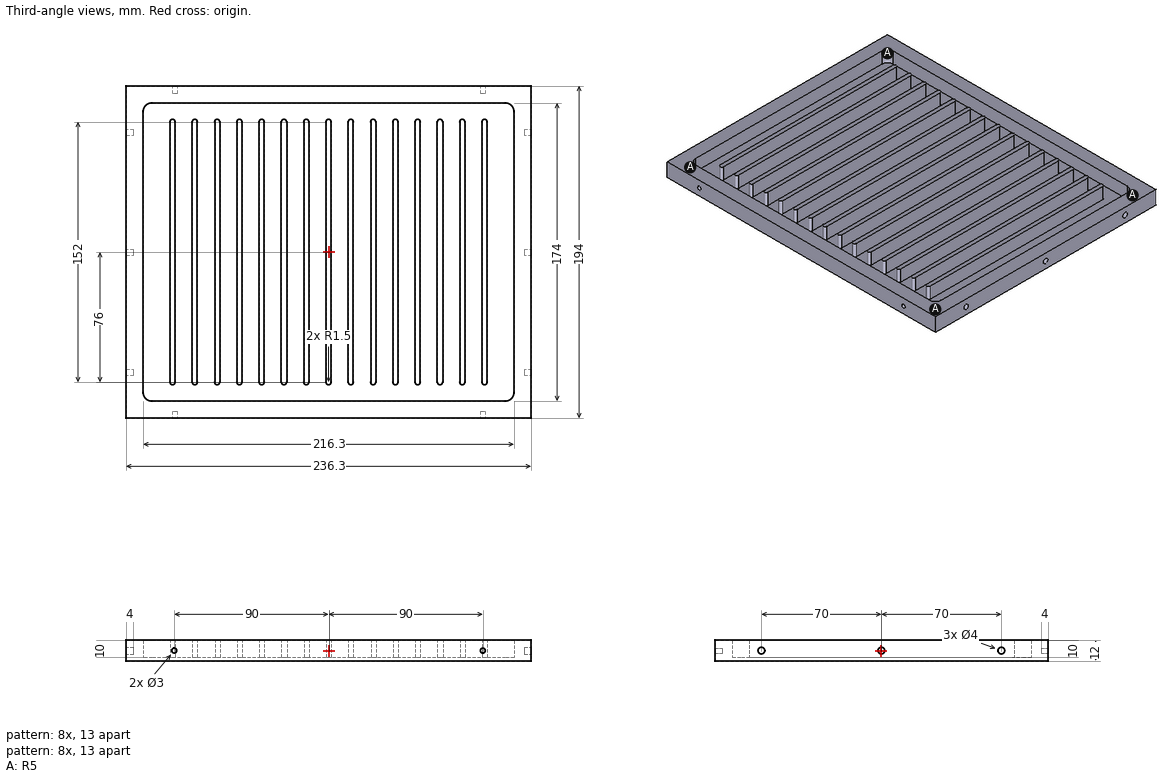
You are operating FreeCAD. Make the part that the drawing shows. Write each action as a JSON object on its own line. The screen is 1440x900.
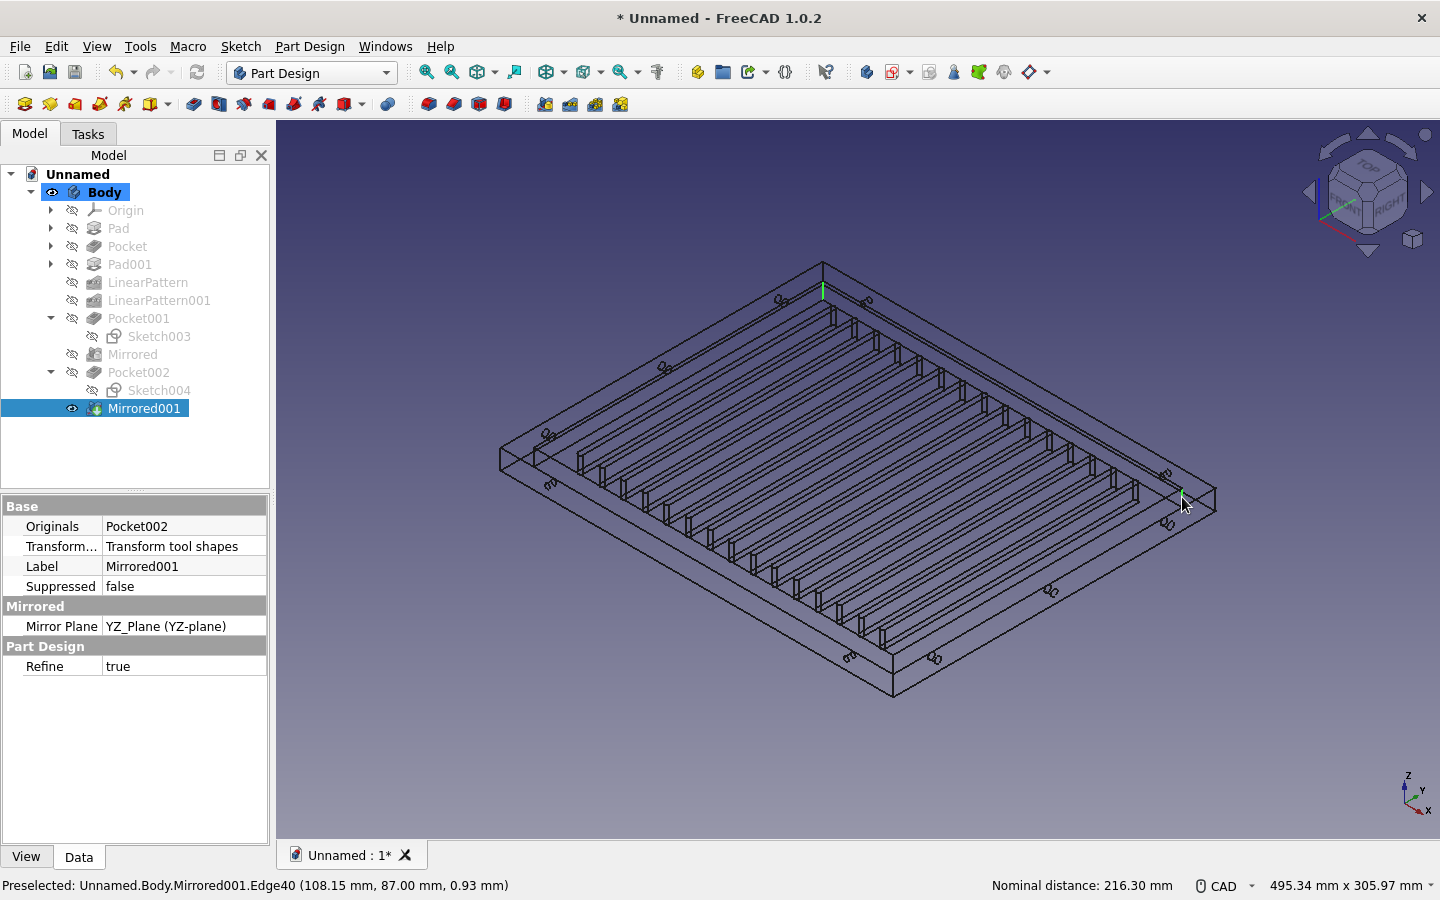
{"action": "left_click", "coordinate": [893, 664], "text": "ctrl"}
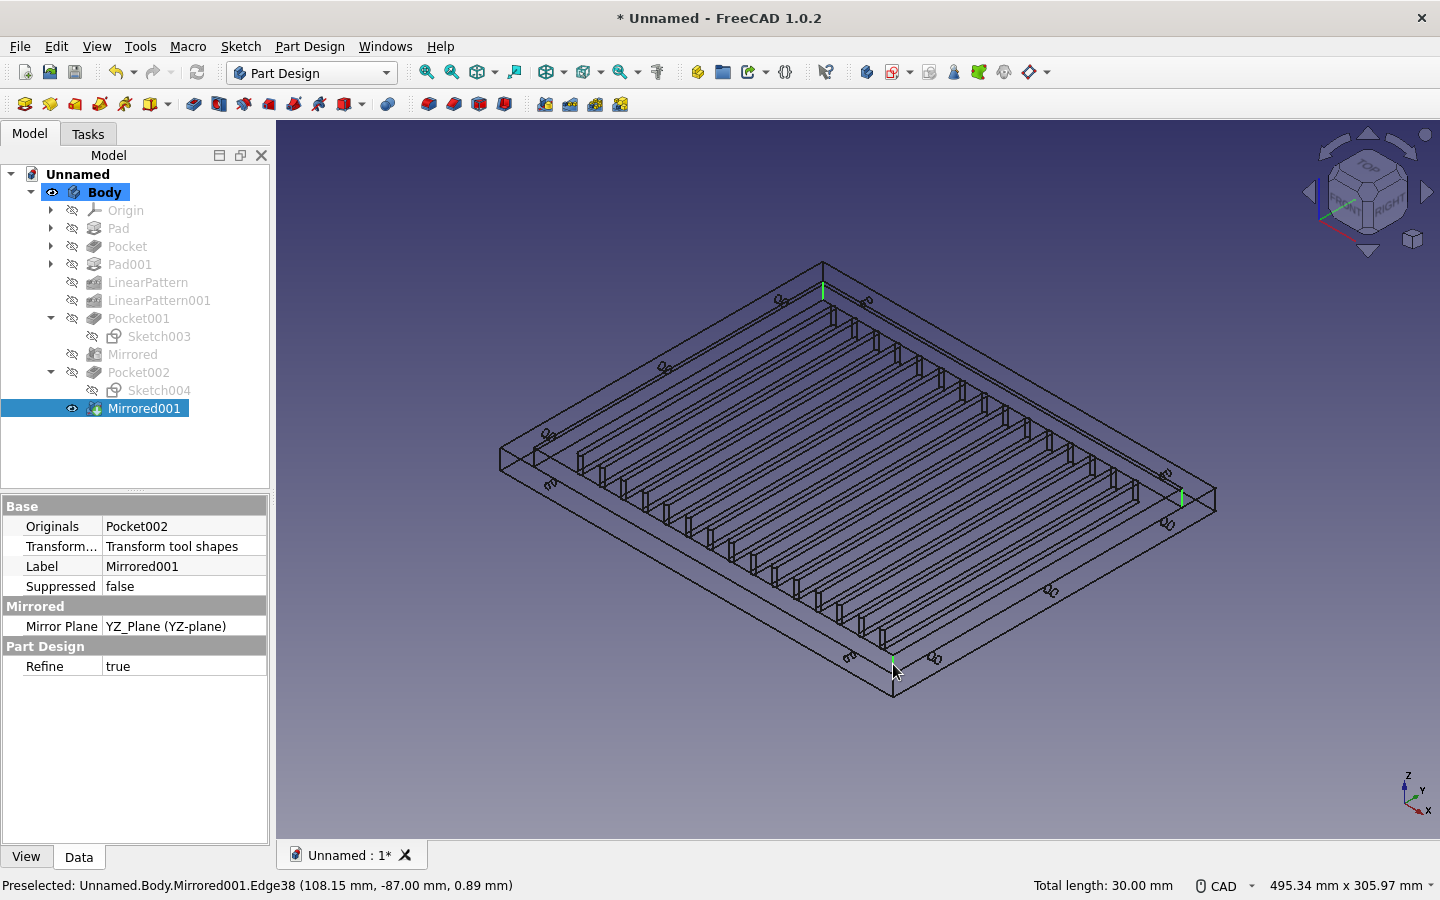
{"action": "left_click", "coordinate": [534, 456], "text": "ctrl"}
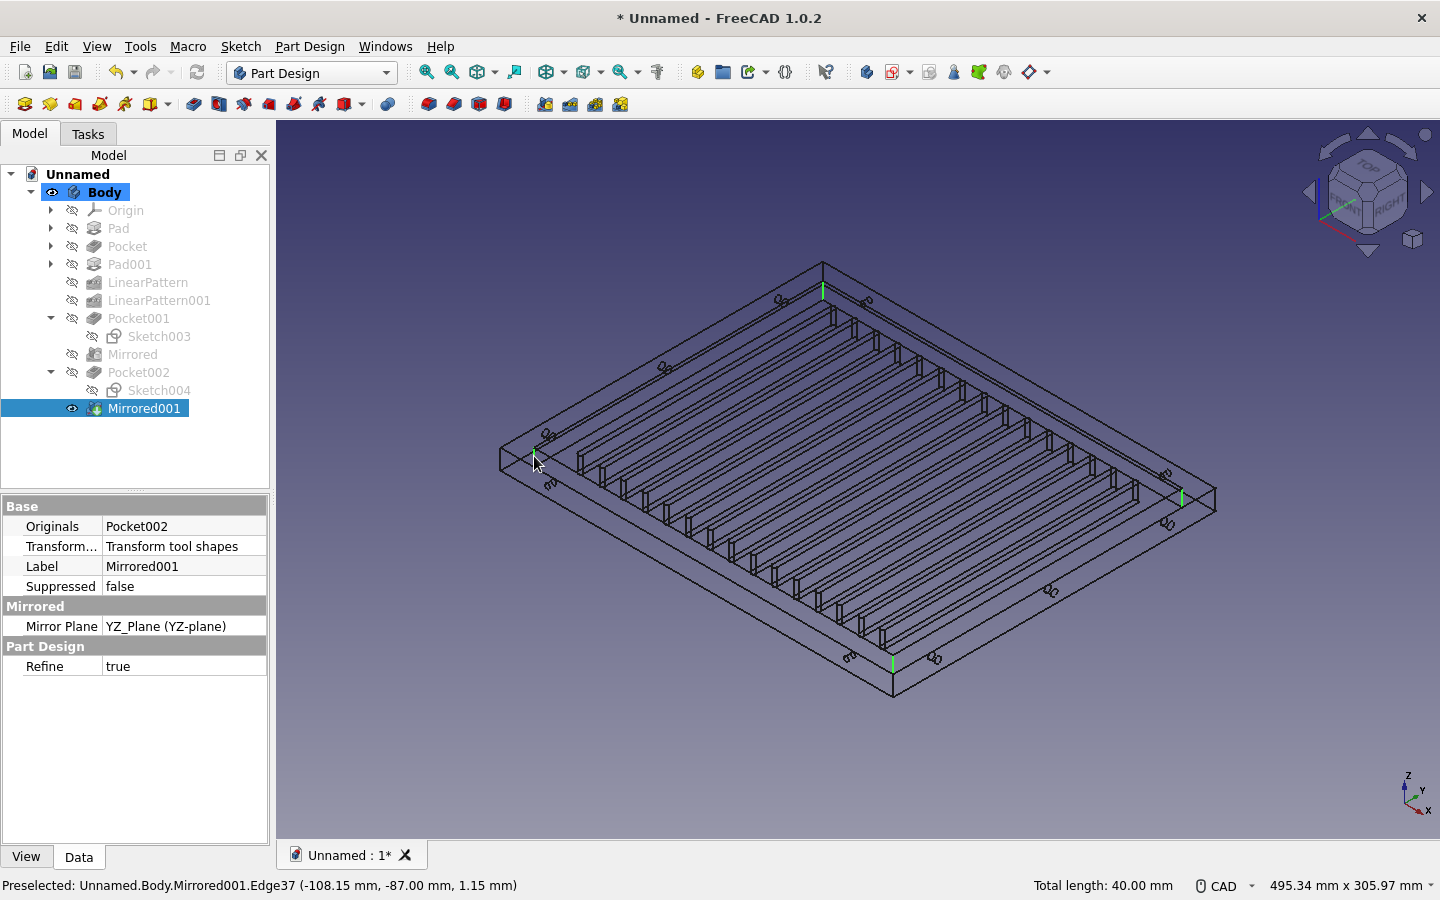
{"action": "key", "text": "v 1"}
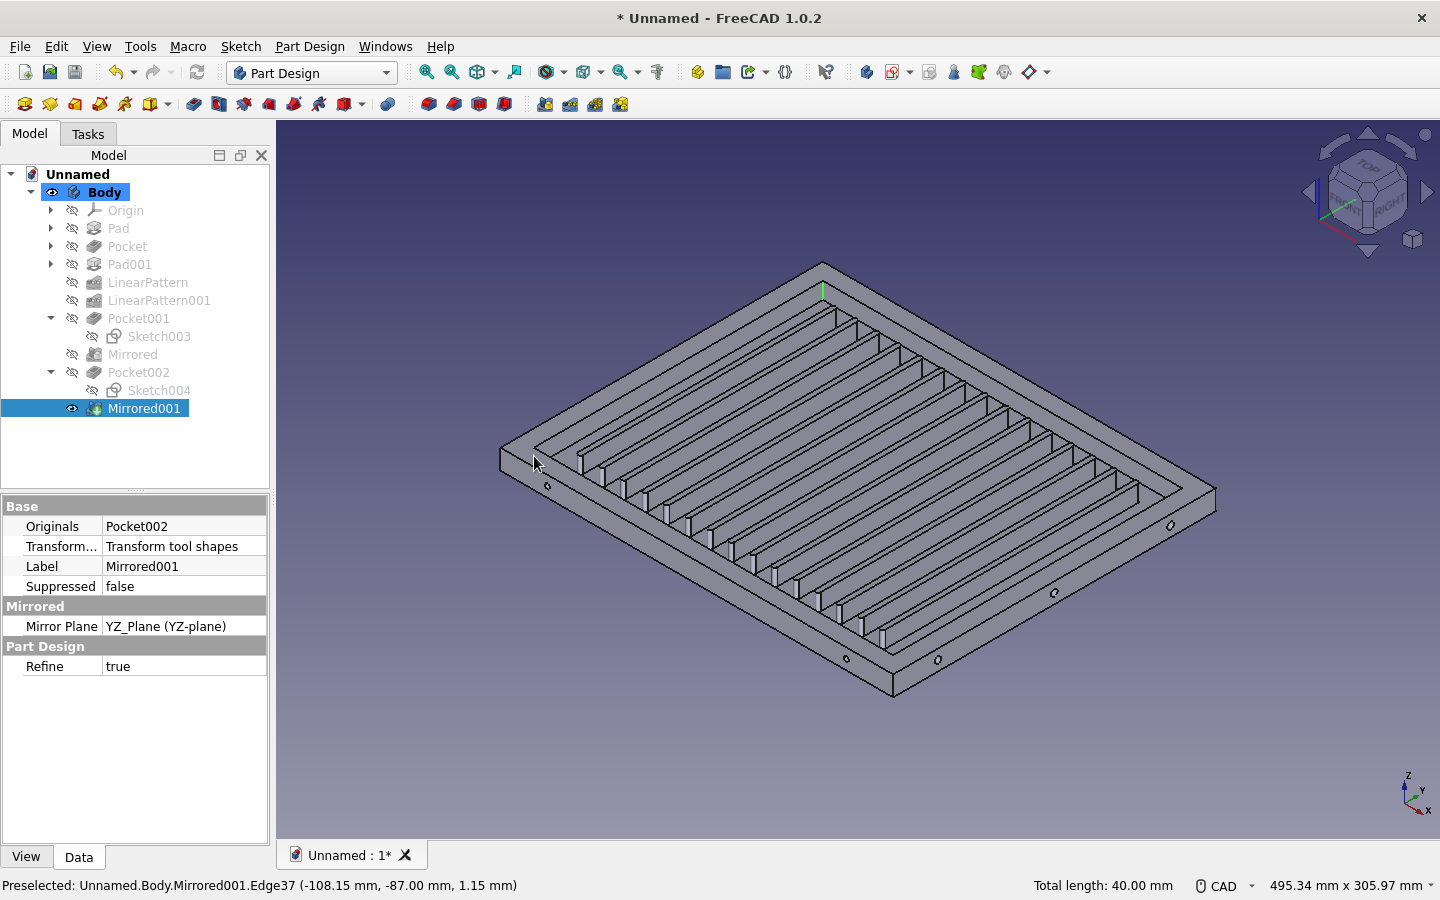
{"action": "left_click", "coordinate": [429, 104]}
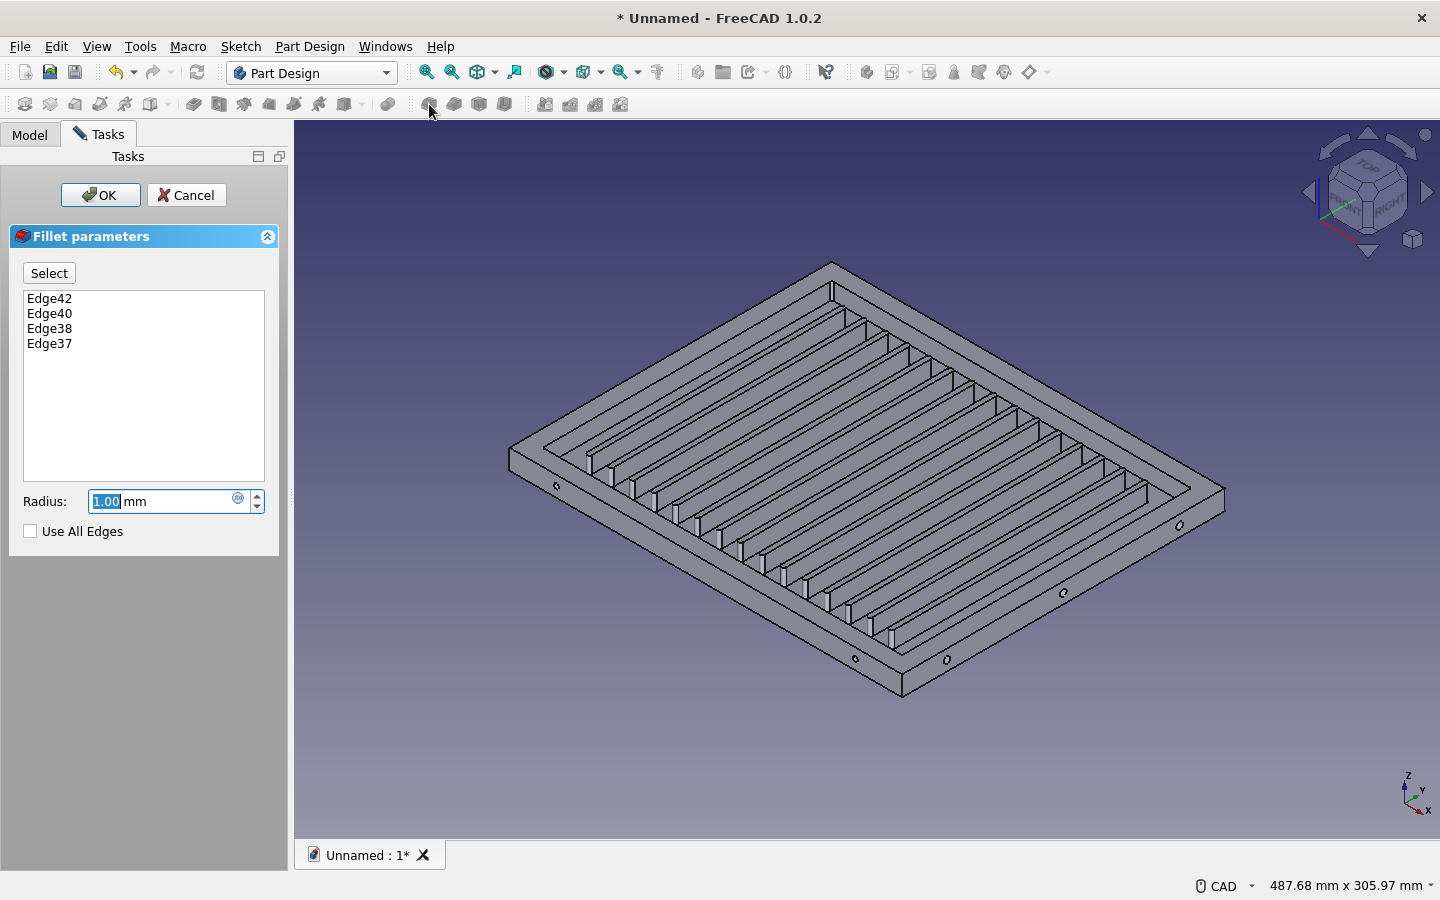
{"action": "type", "text": "5"}
{"action": "key", "text": "Tab"}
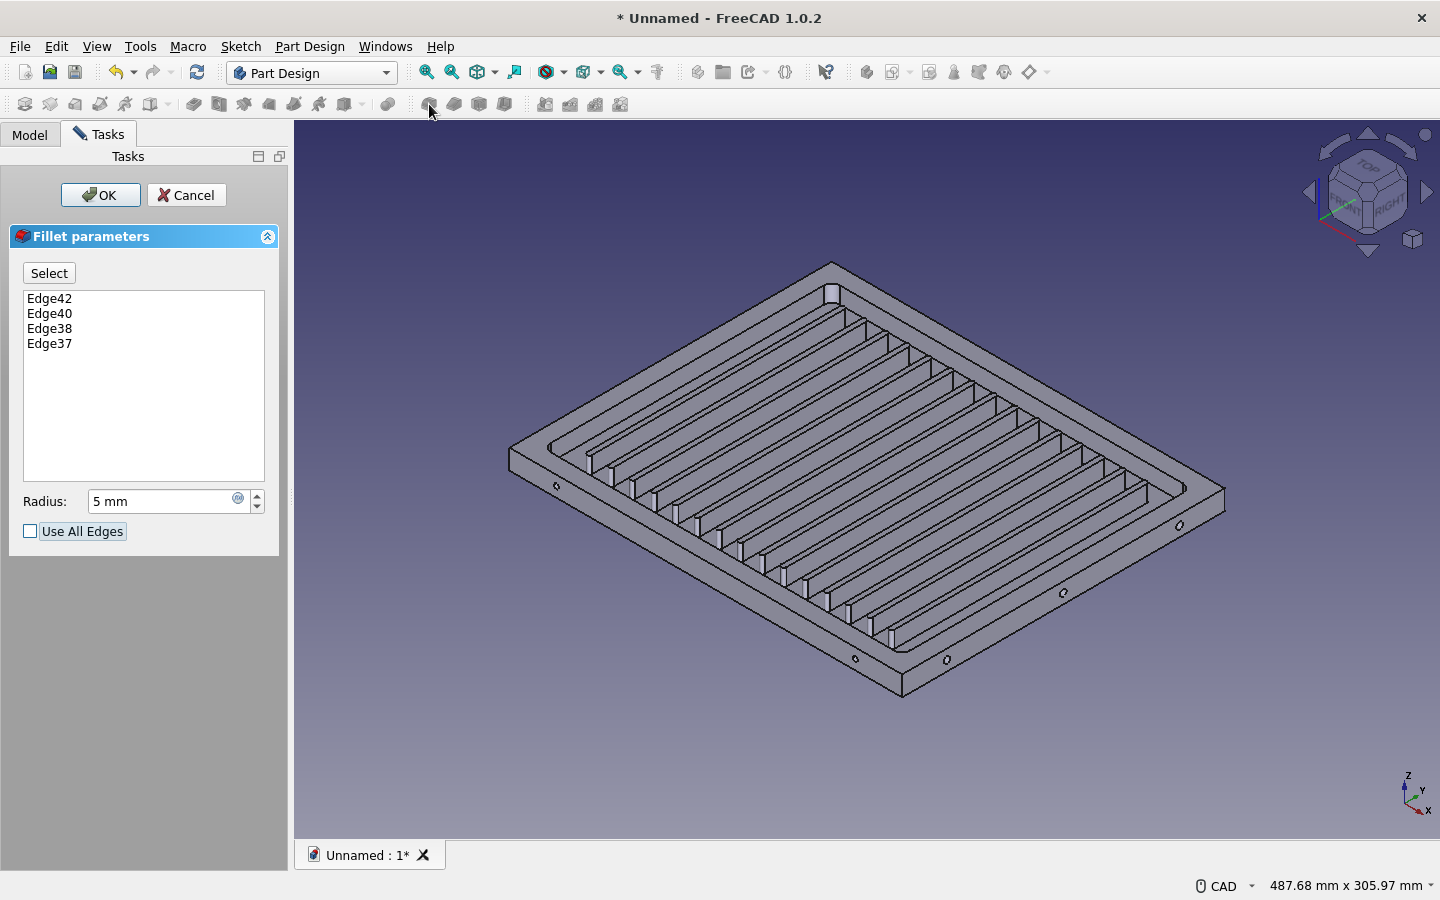
{"action": "left_click", "coordinate": [101, 195]}